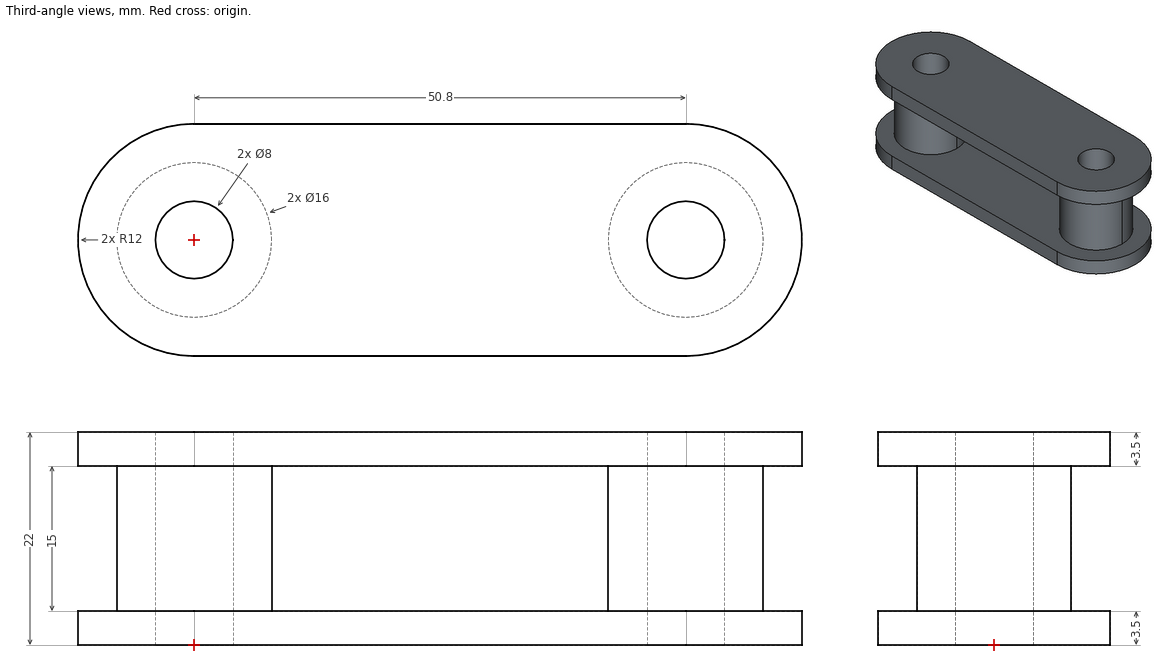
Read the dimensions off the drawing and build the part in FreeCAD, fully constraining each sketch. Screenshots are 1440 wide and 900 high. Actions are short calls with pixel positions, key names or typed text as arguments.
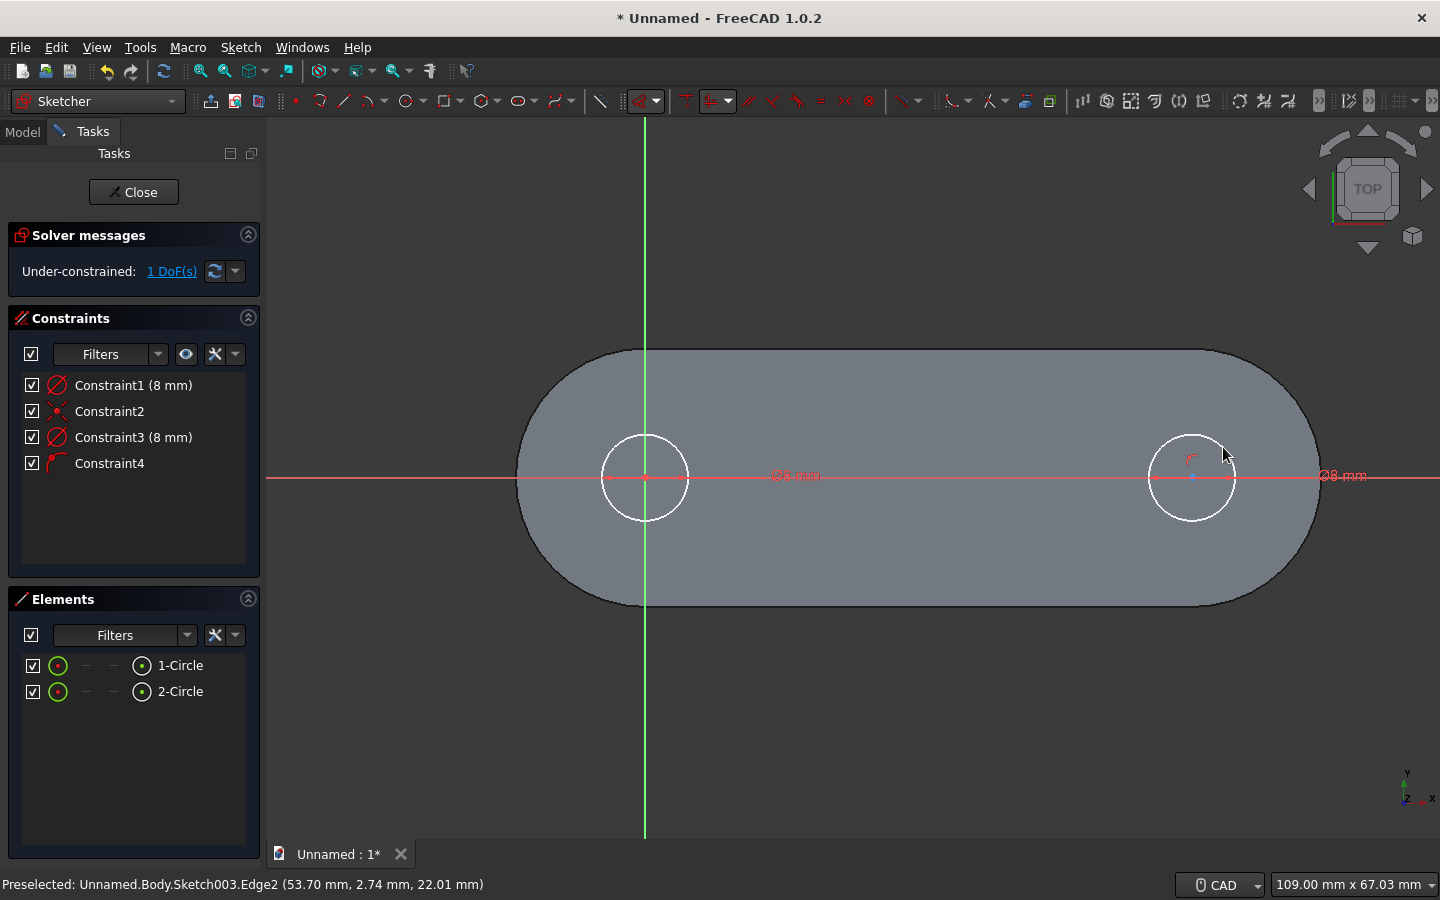
click(1192, 478)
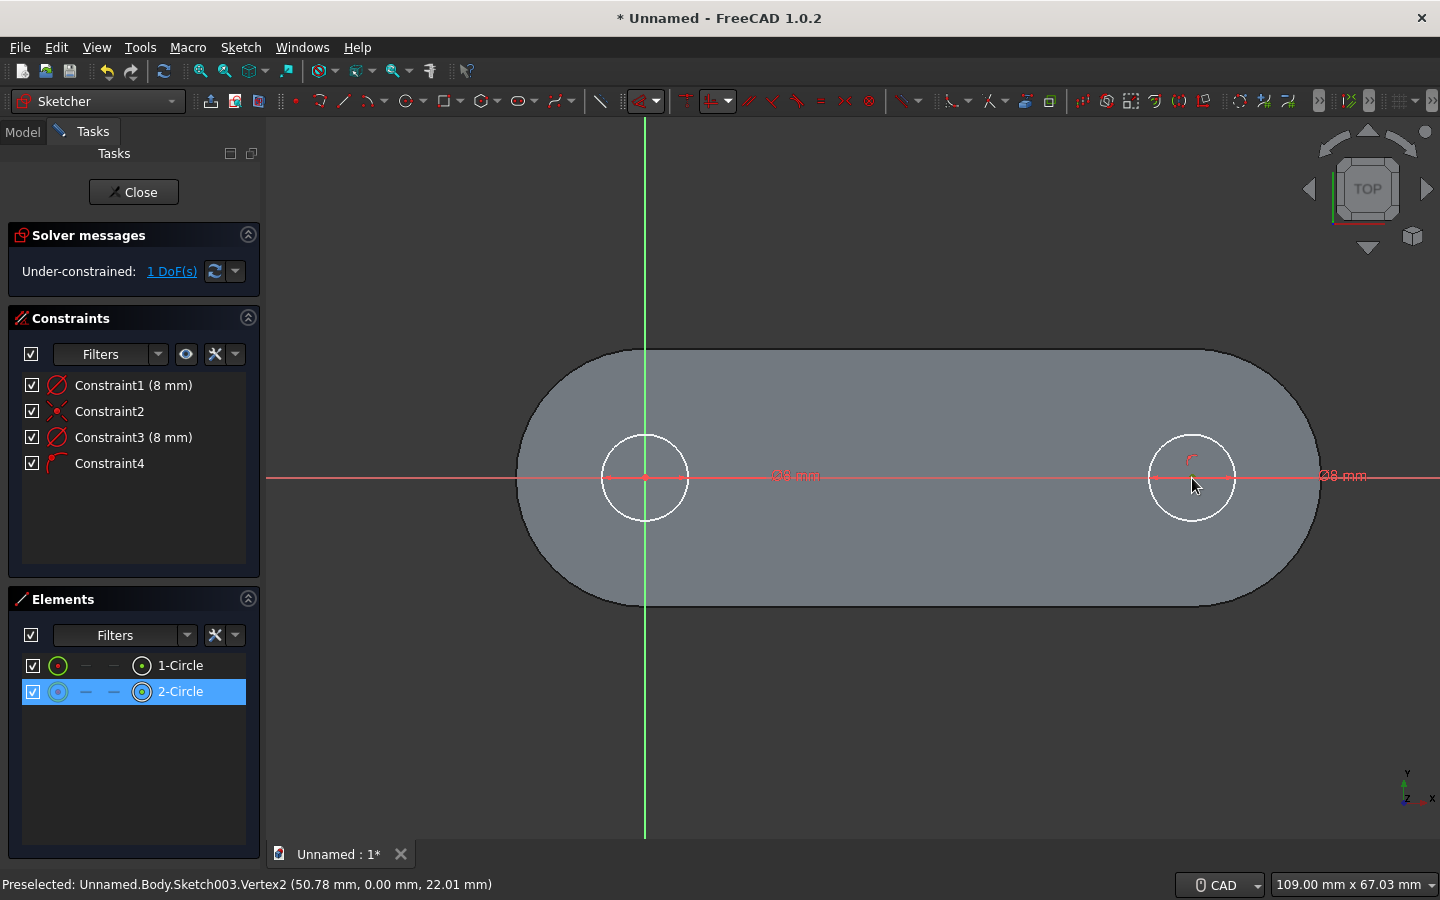
click(658, 102)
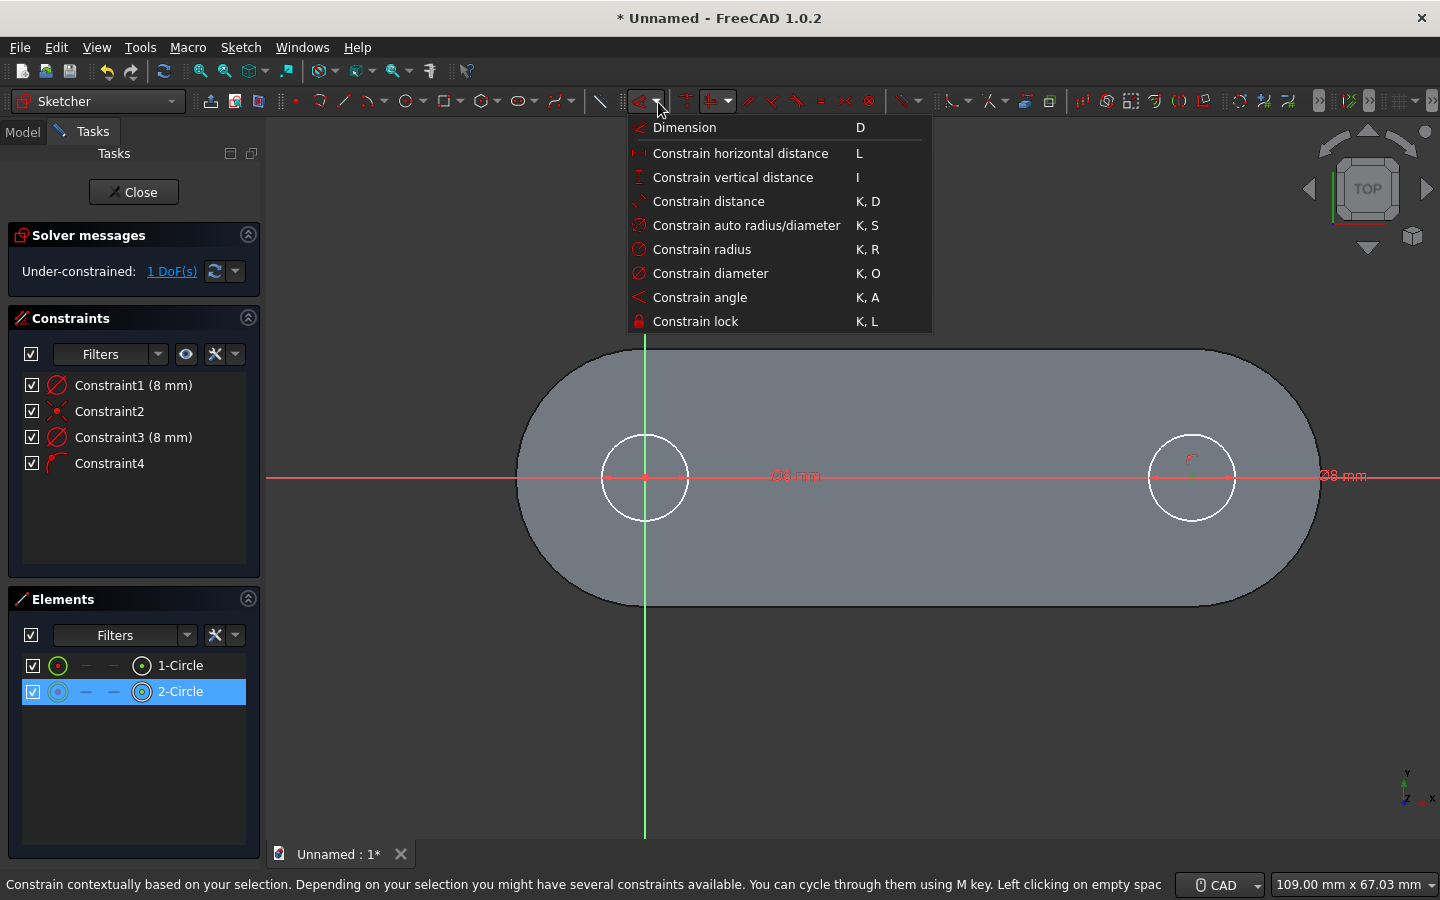
click(780, 153)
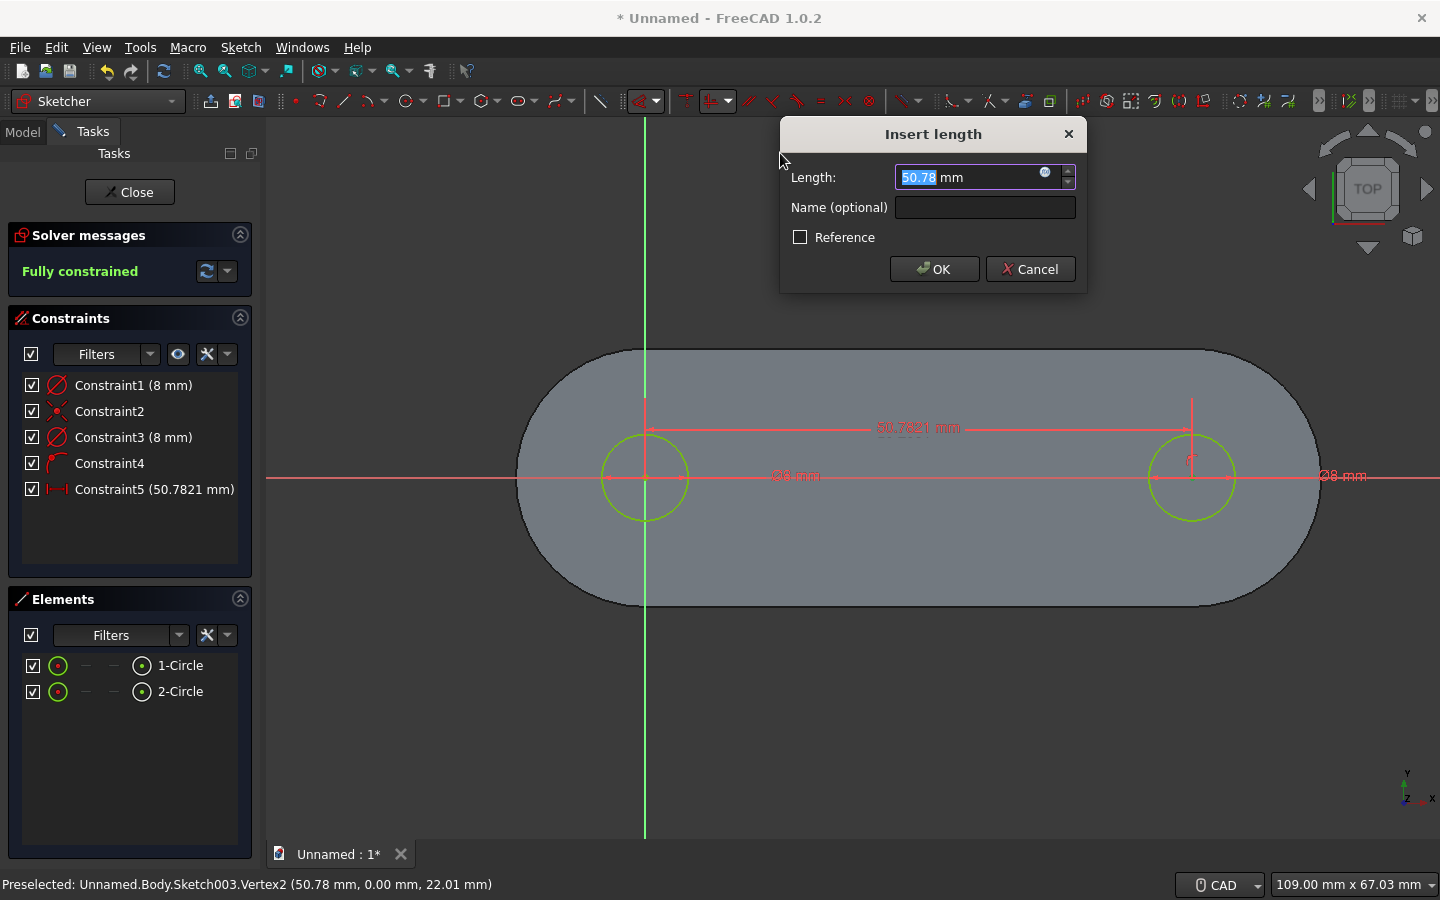
text(50.8)
key(Return)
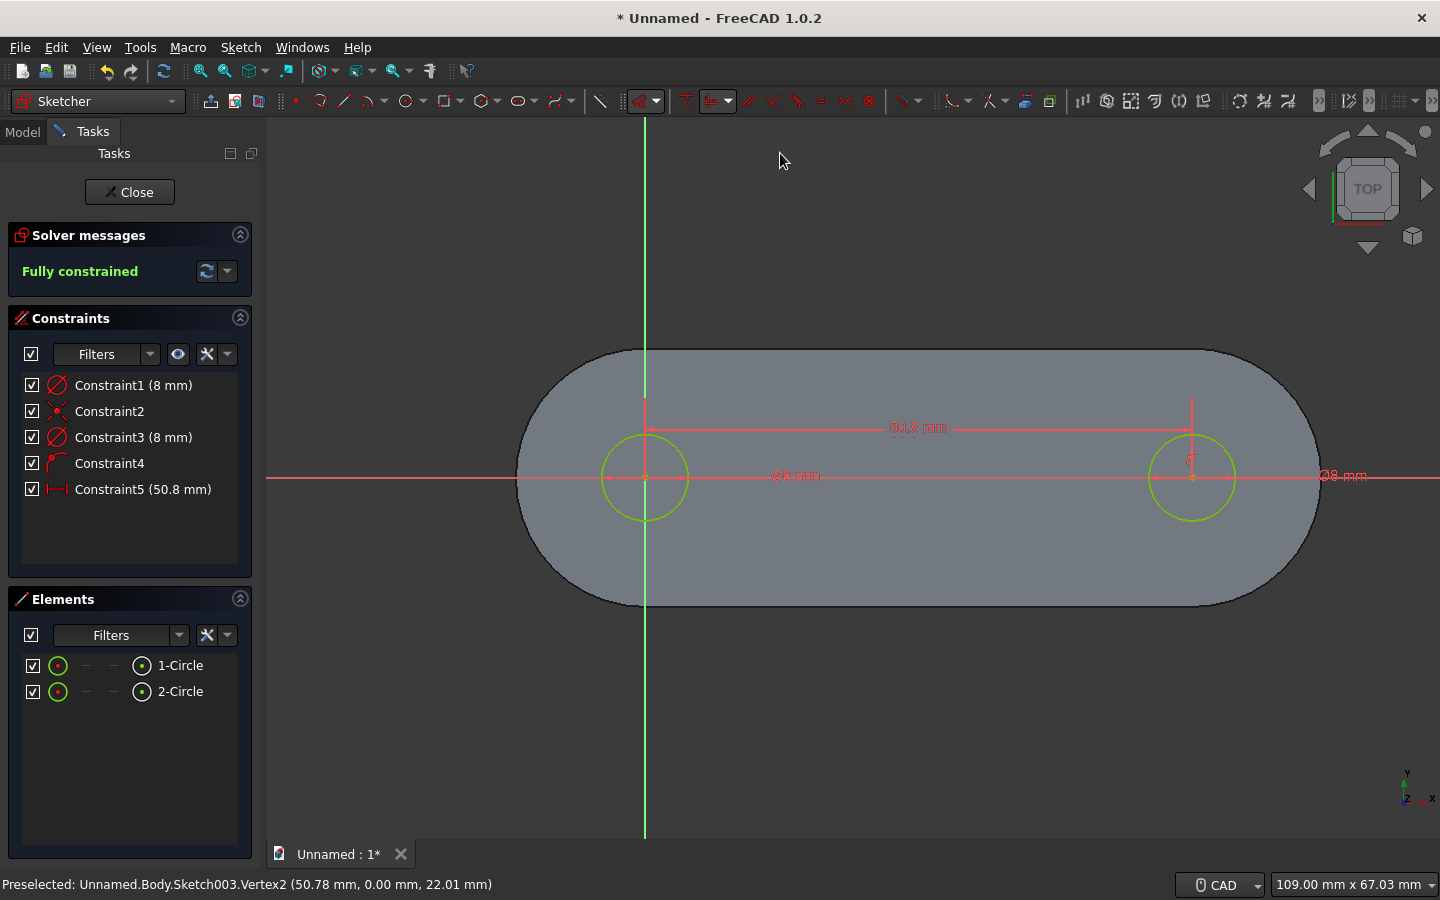
click(130, 192)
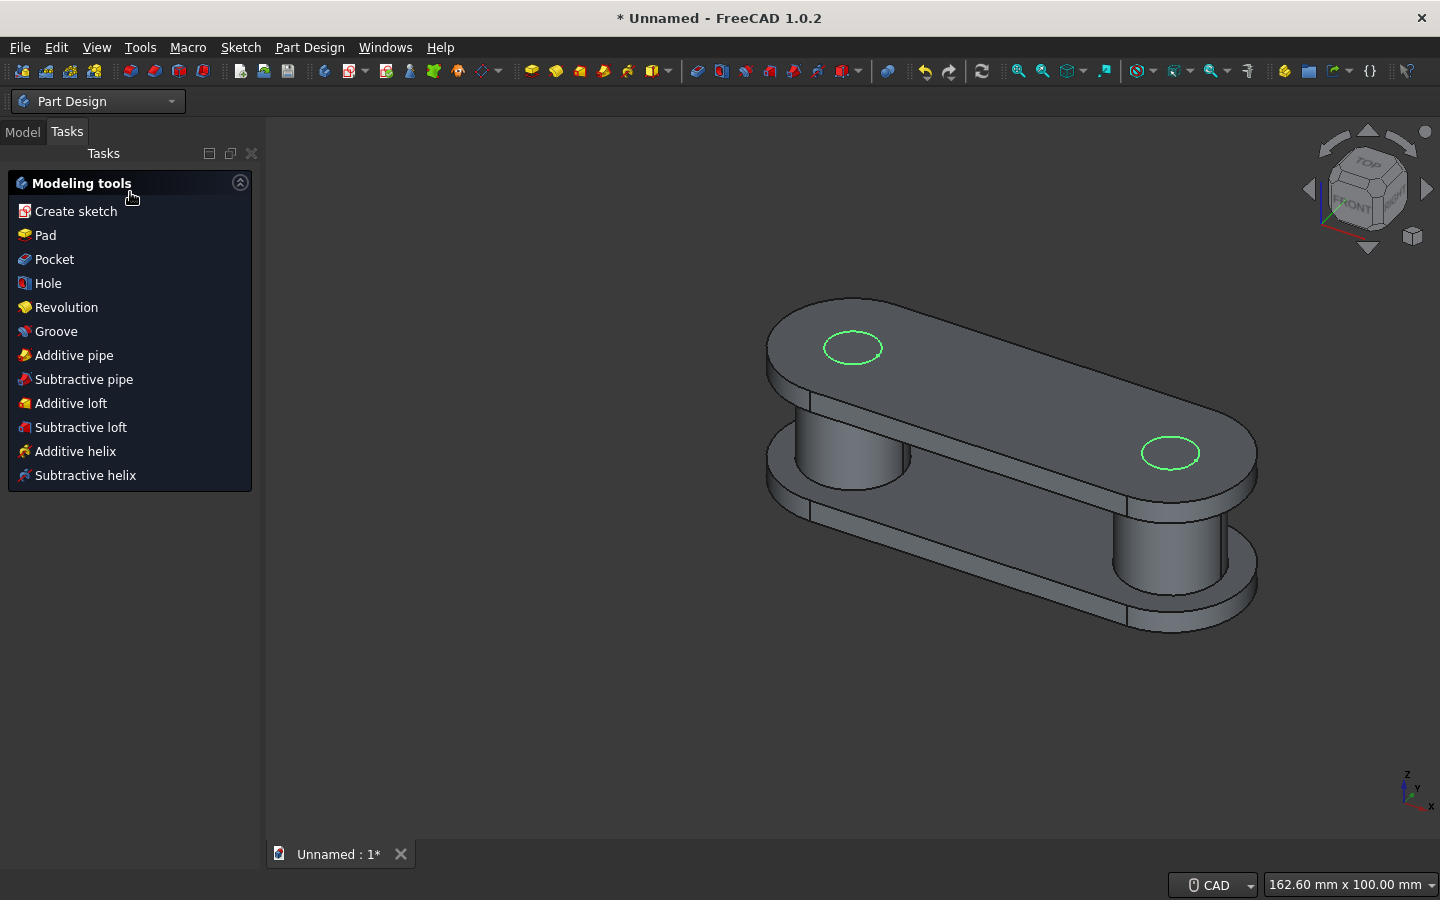
click(698, 72)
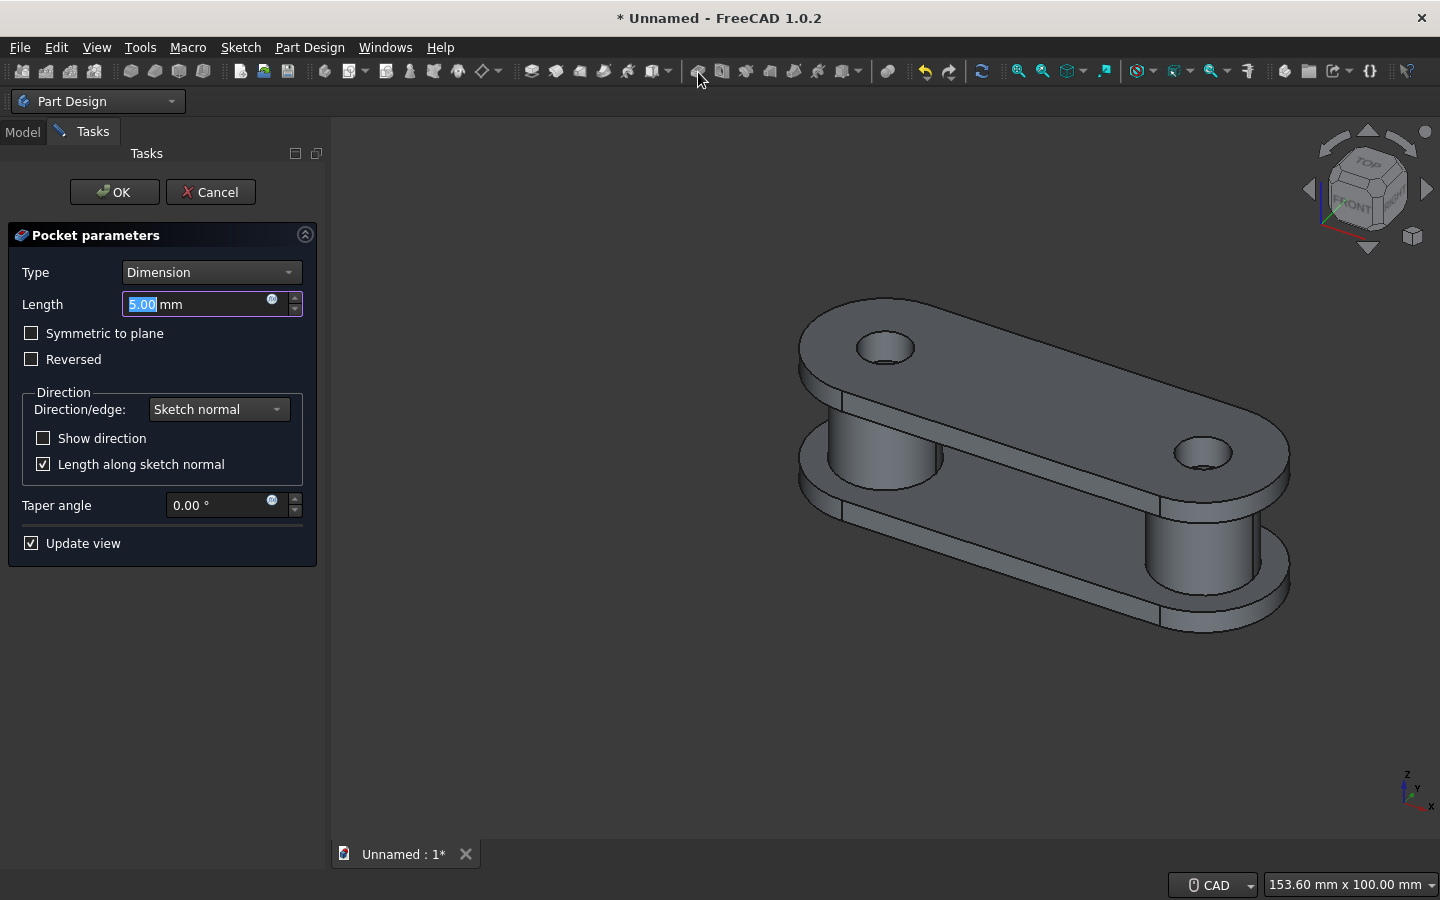
text(22)
key(Tab)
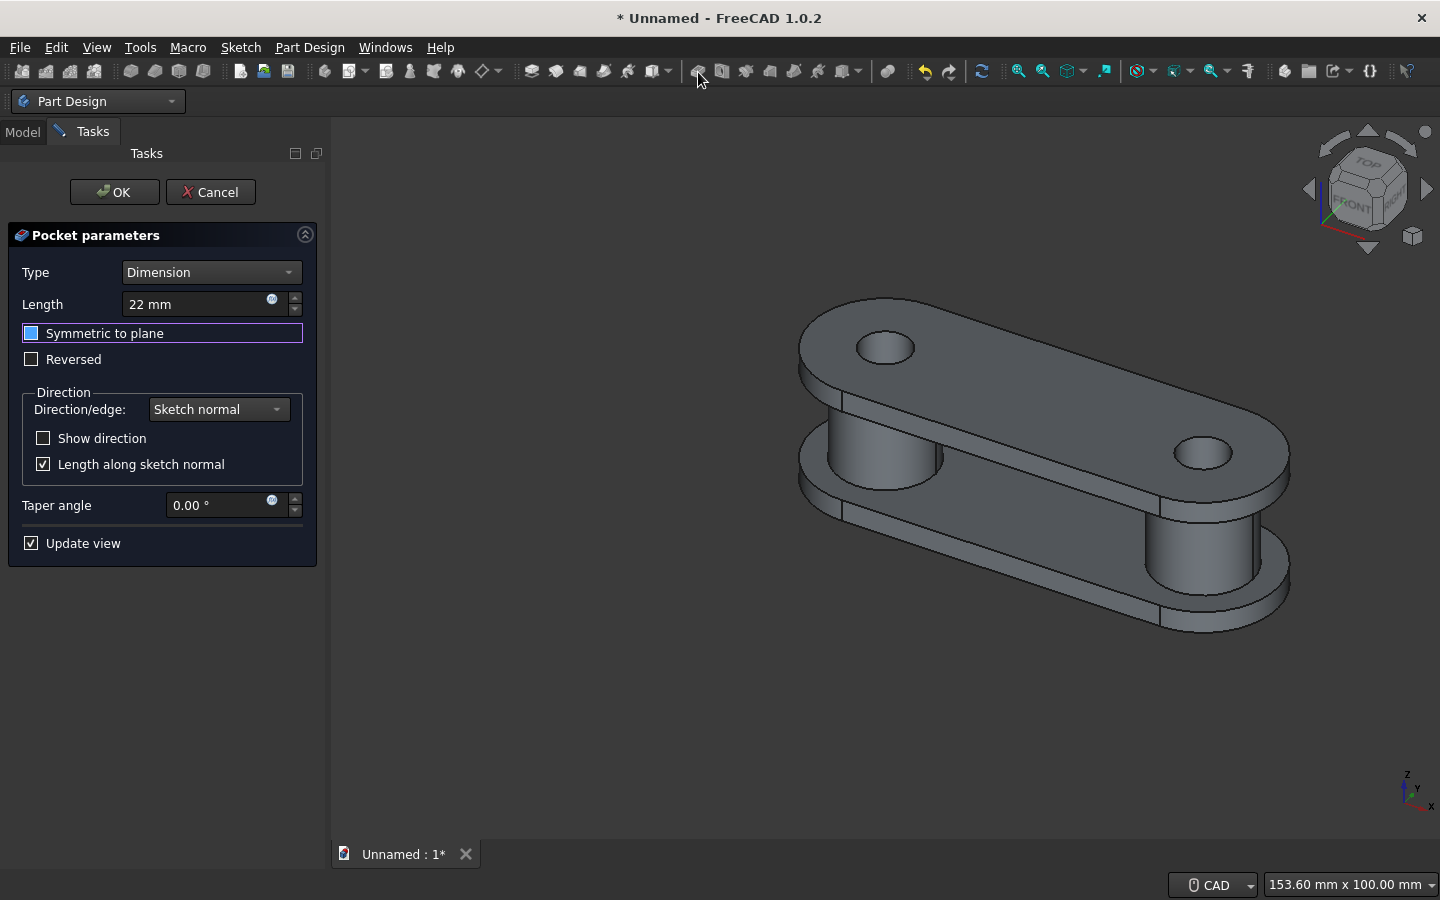
click(115, 192)